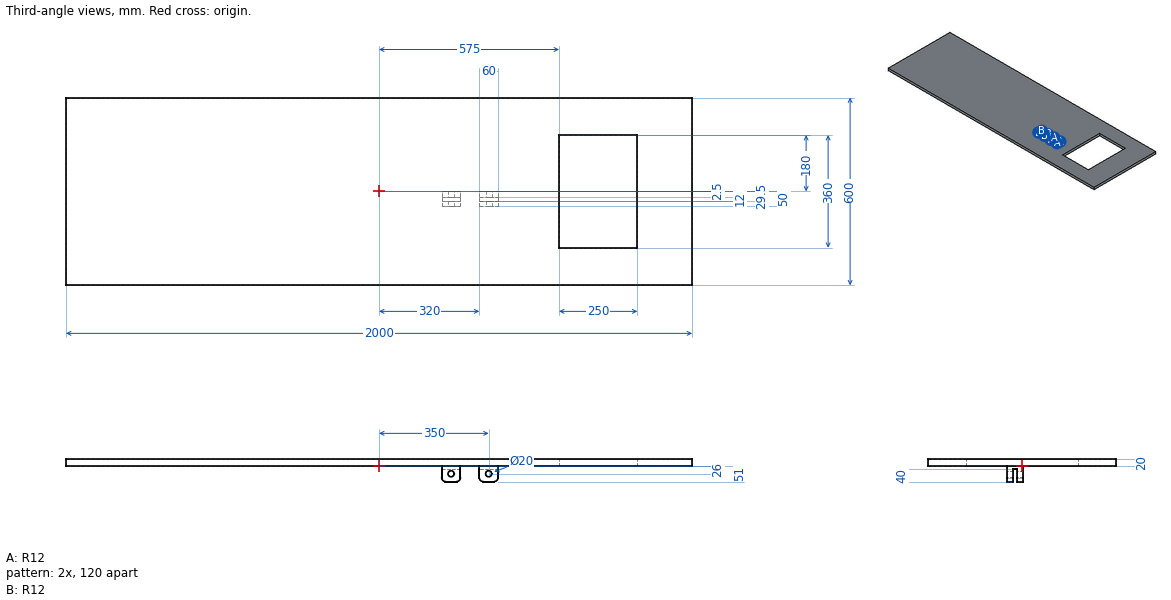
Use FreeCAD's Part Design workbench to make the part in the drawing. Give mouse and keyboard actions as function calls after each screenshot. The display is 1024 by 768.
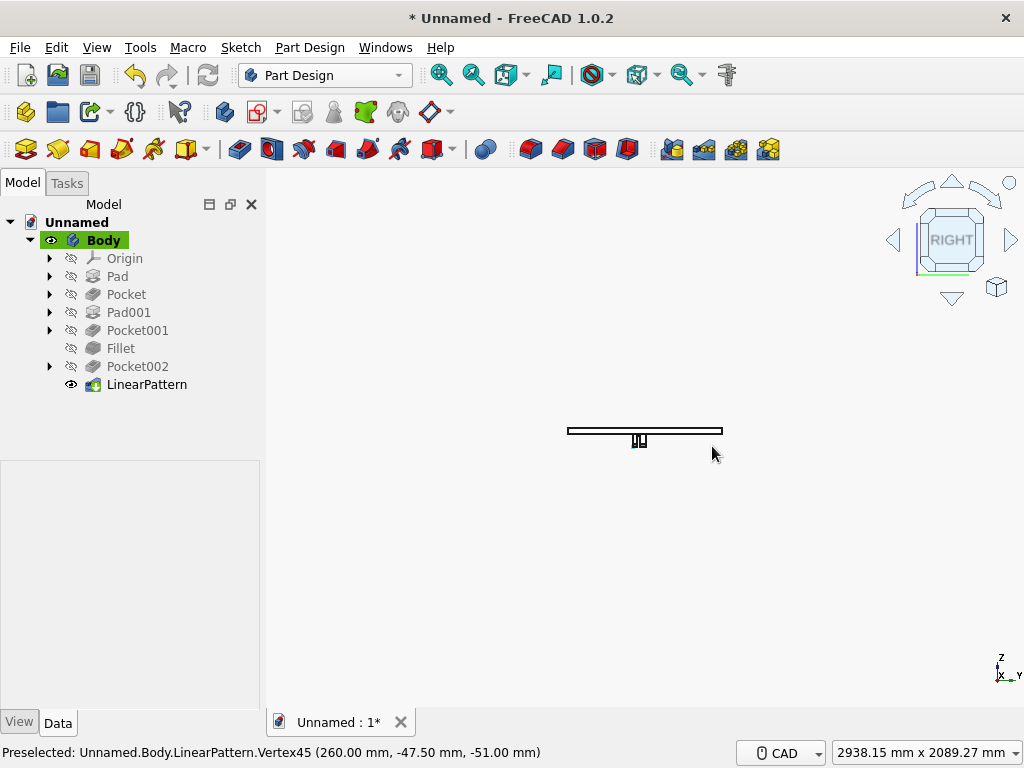
key(v)
key(f)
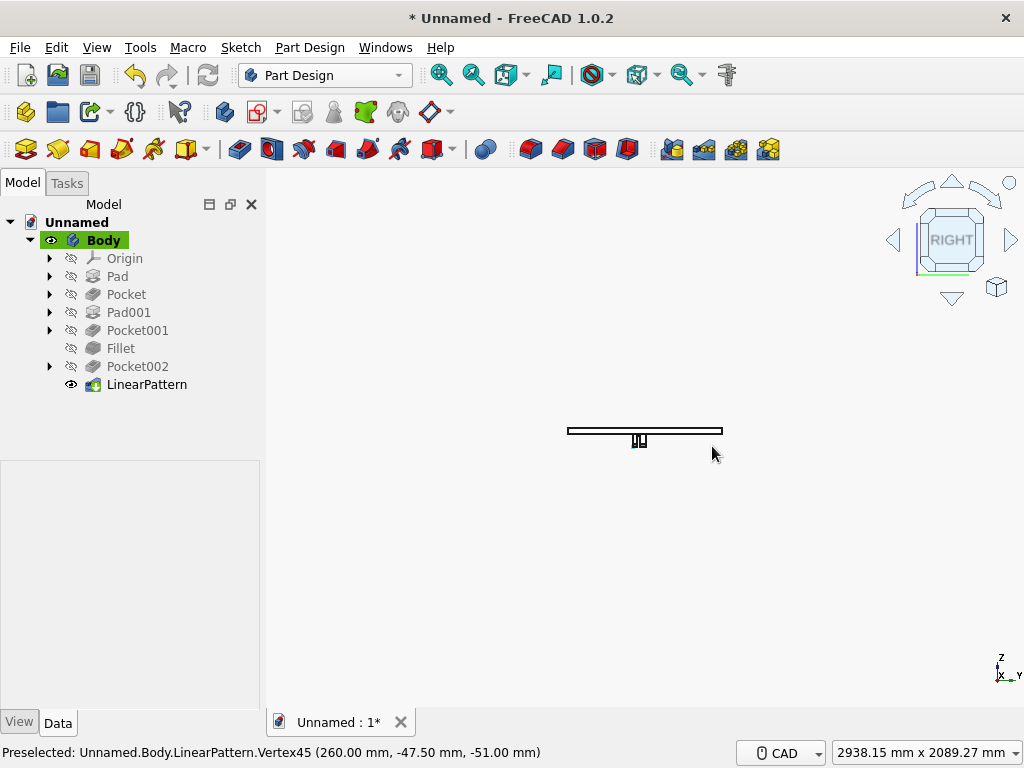
scroll(643, 446, up, 11)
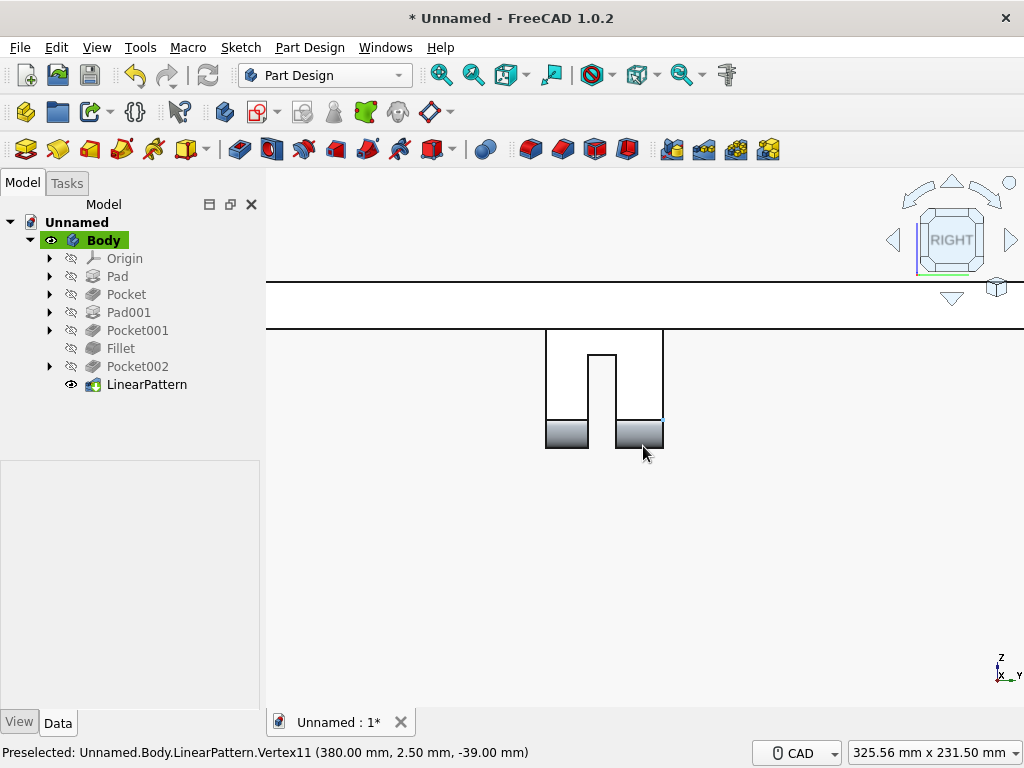
click(442, 76)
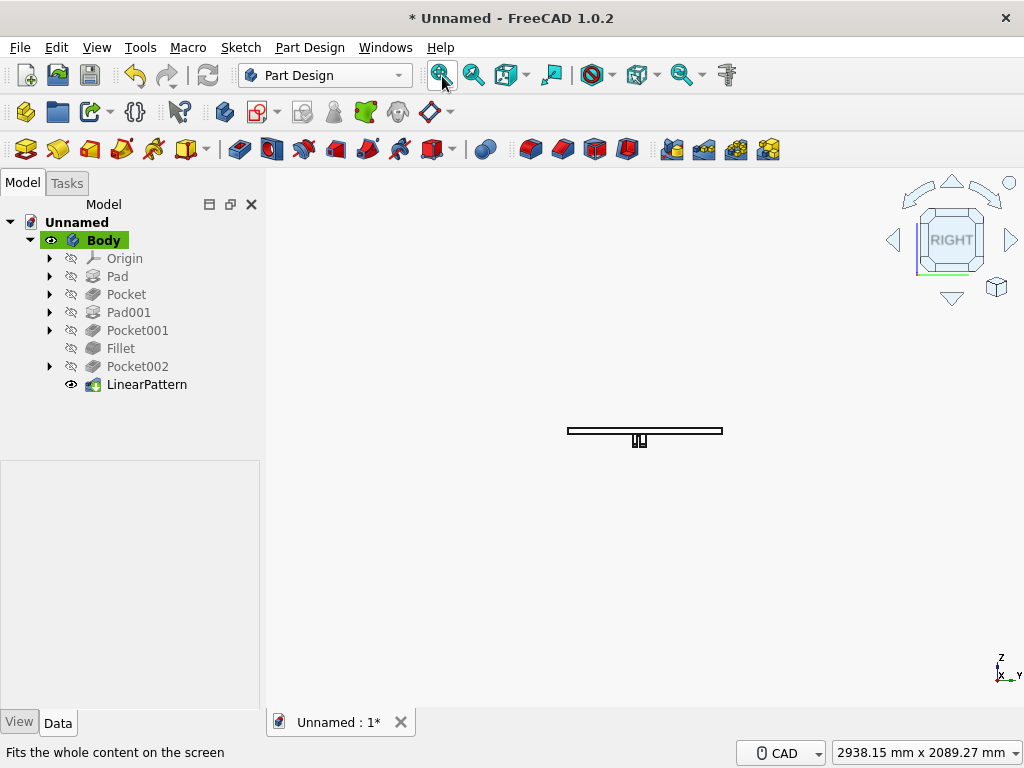
key(5)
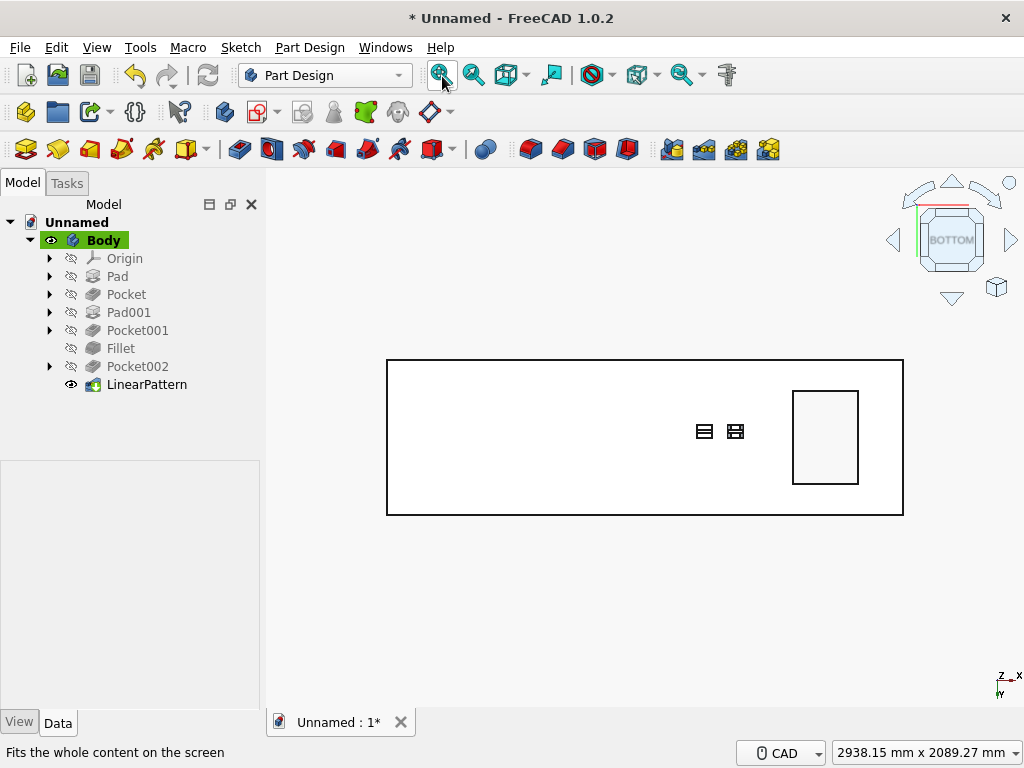
scroll(712, 435, up, 11)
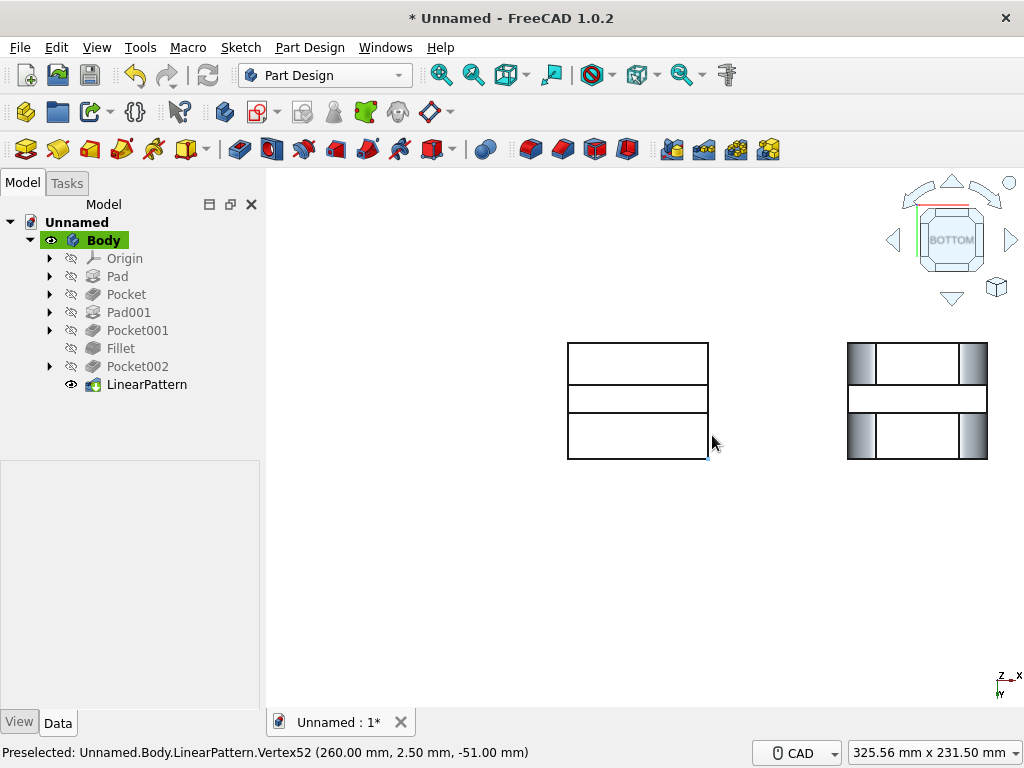
click(708, 435)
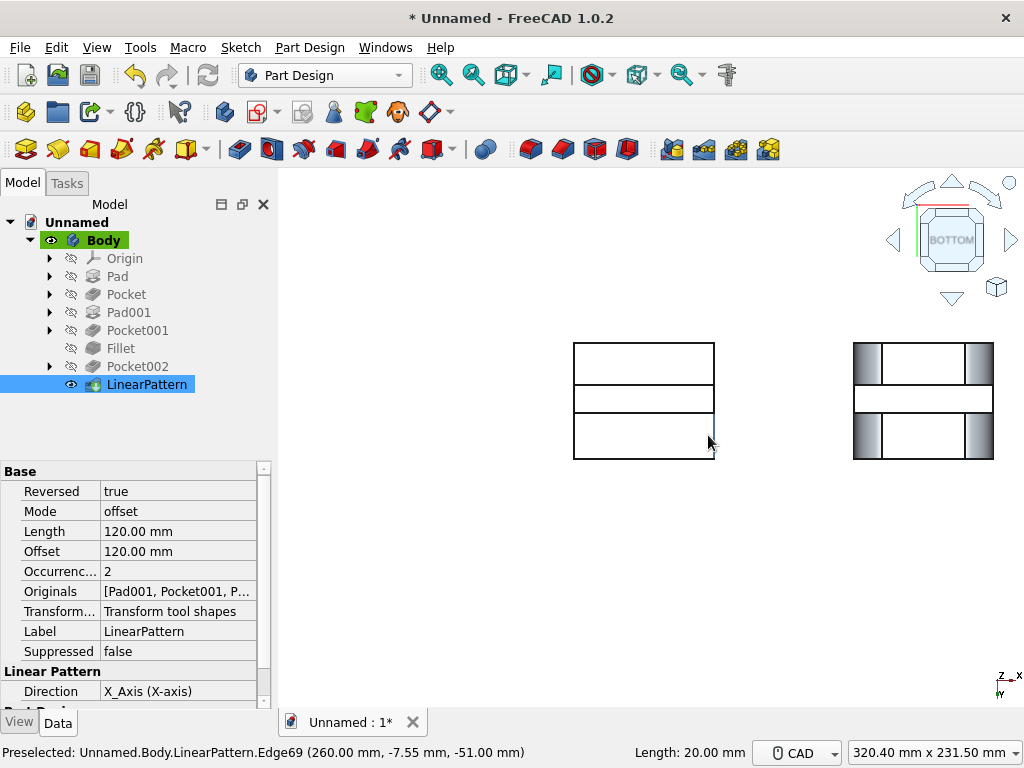
click(574, 363, ctrl)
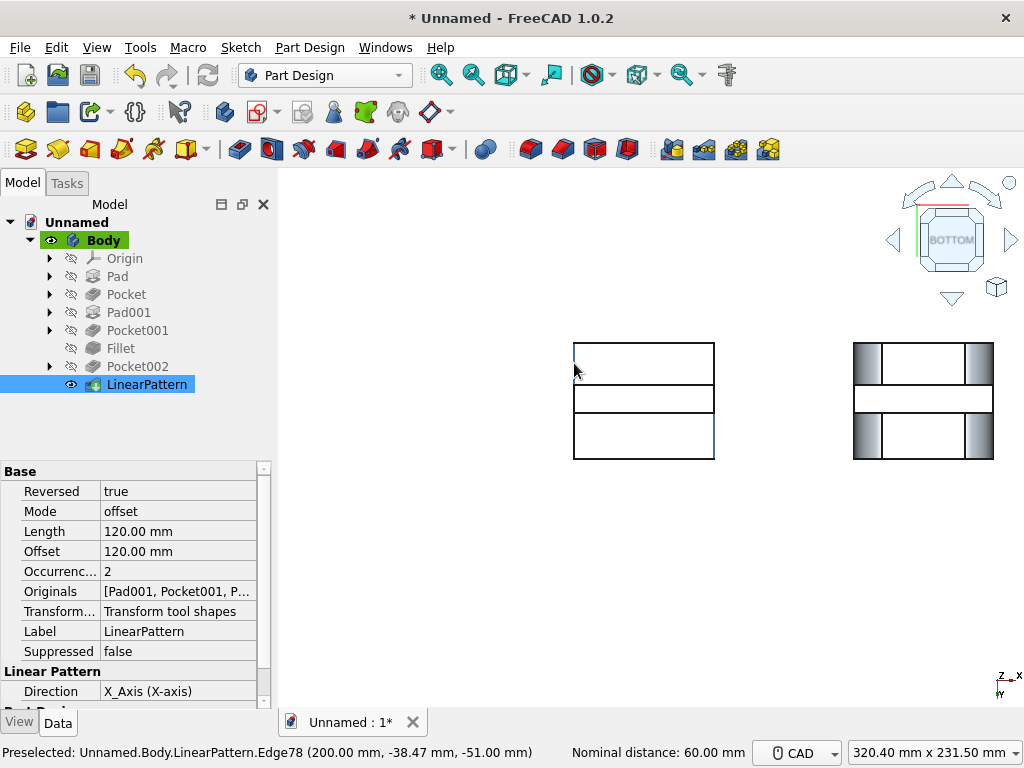
click(714, 363, ctrl)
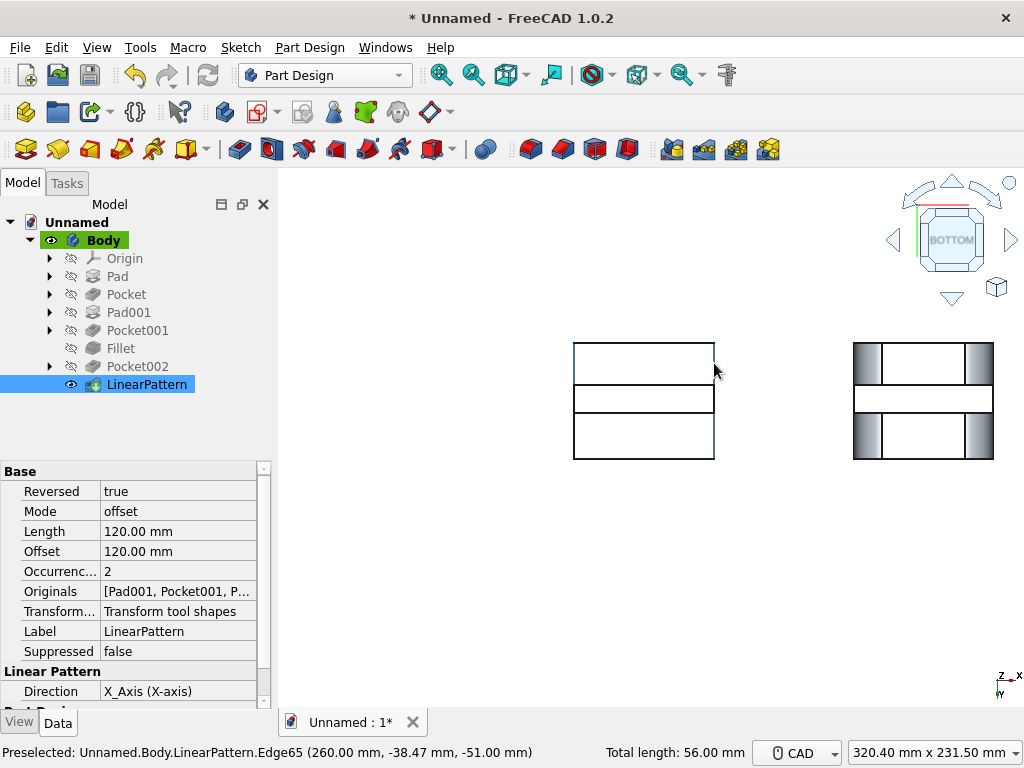
click(574, 435, ctrl)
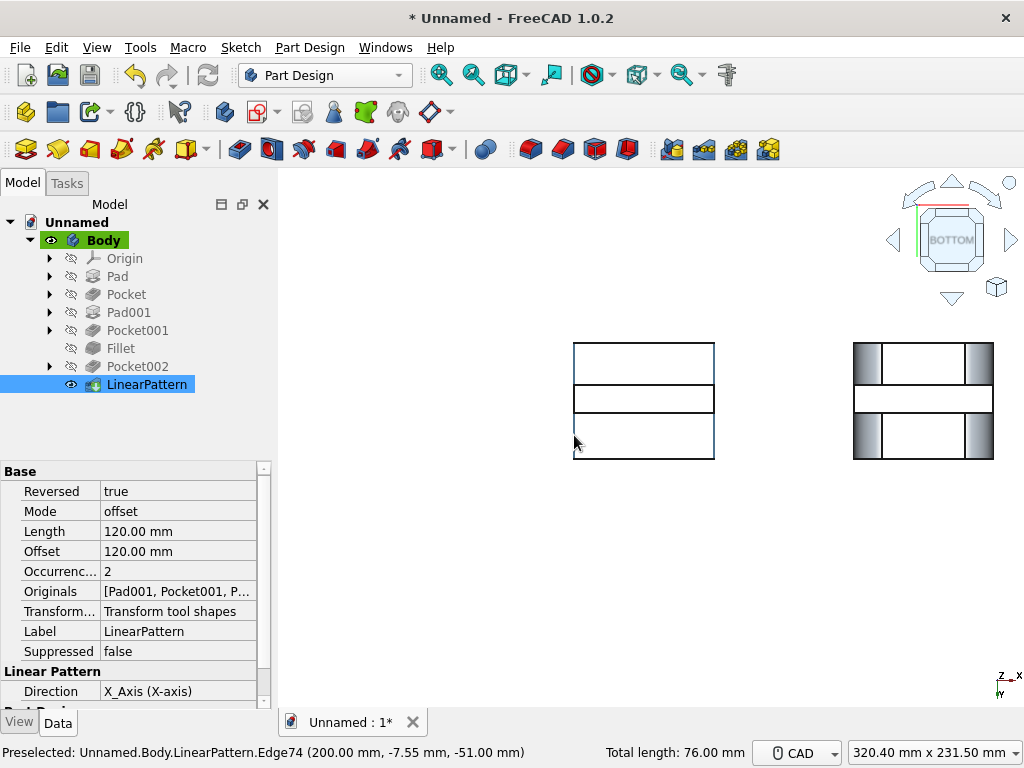
click(532, 150)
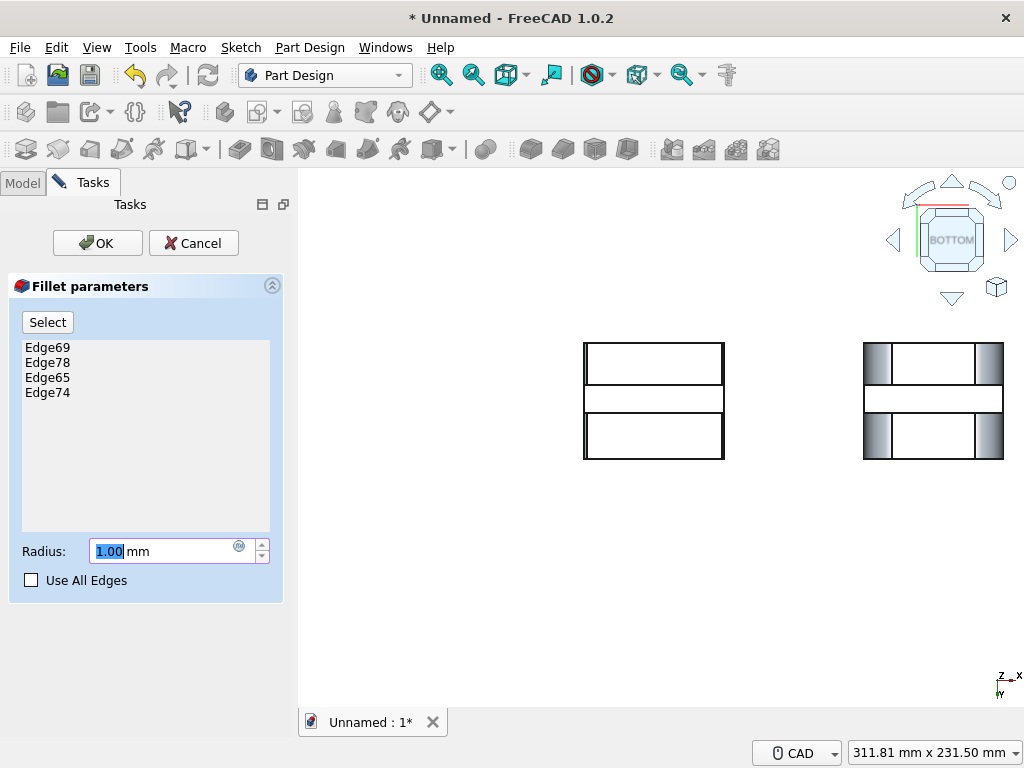
text(12)
key(Tab)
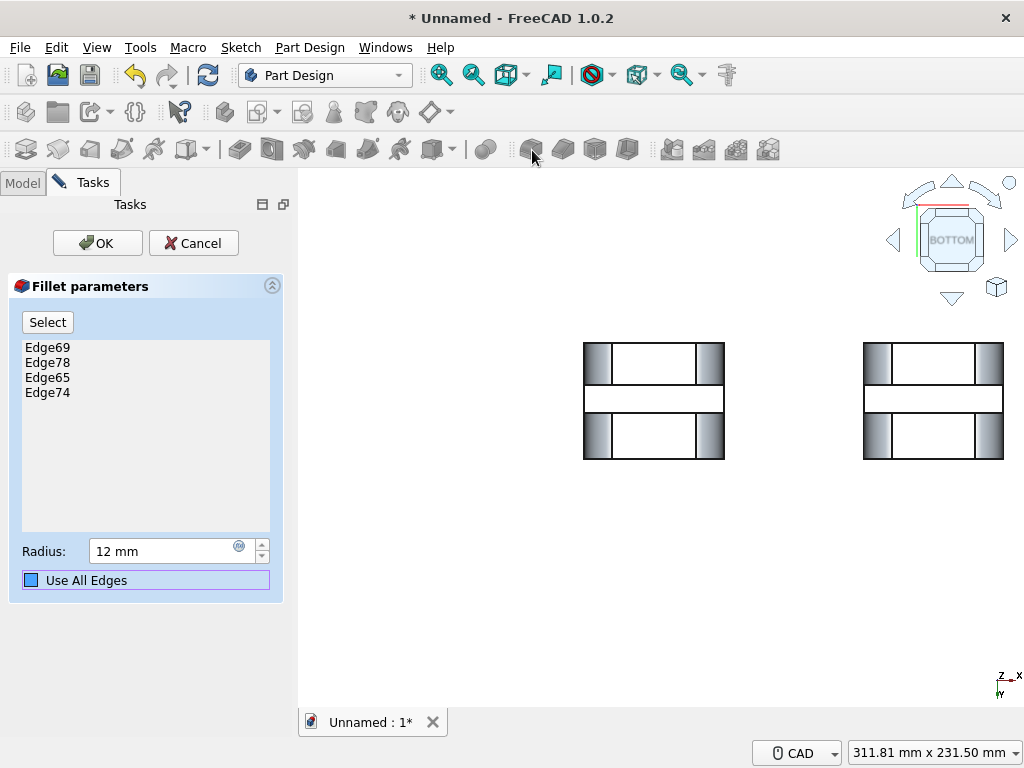
click(98, 243)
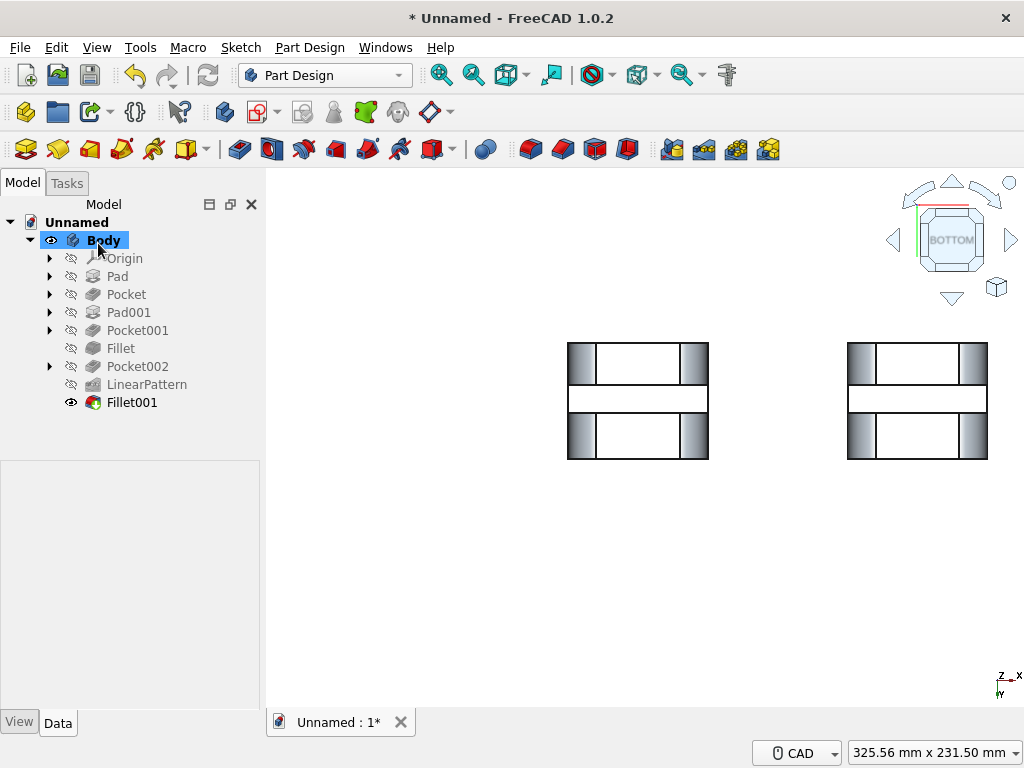
key(0)